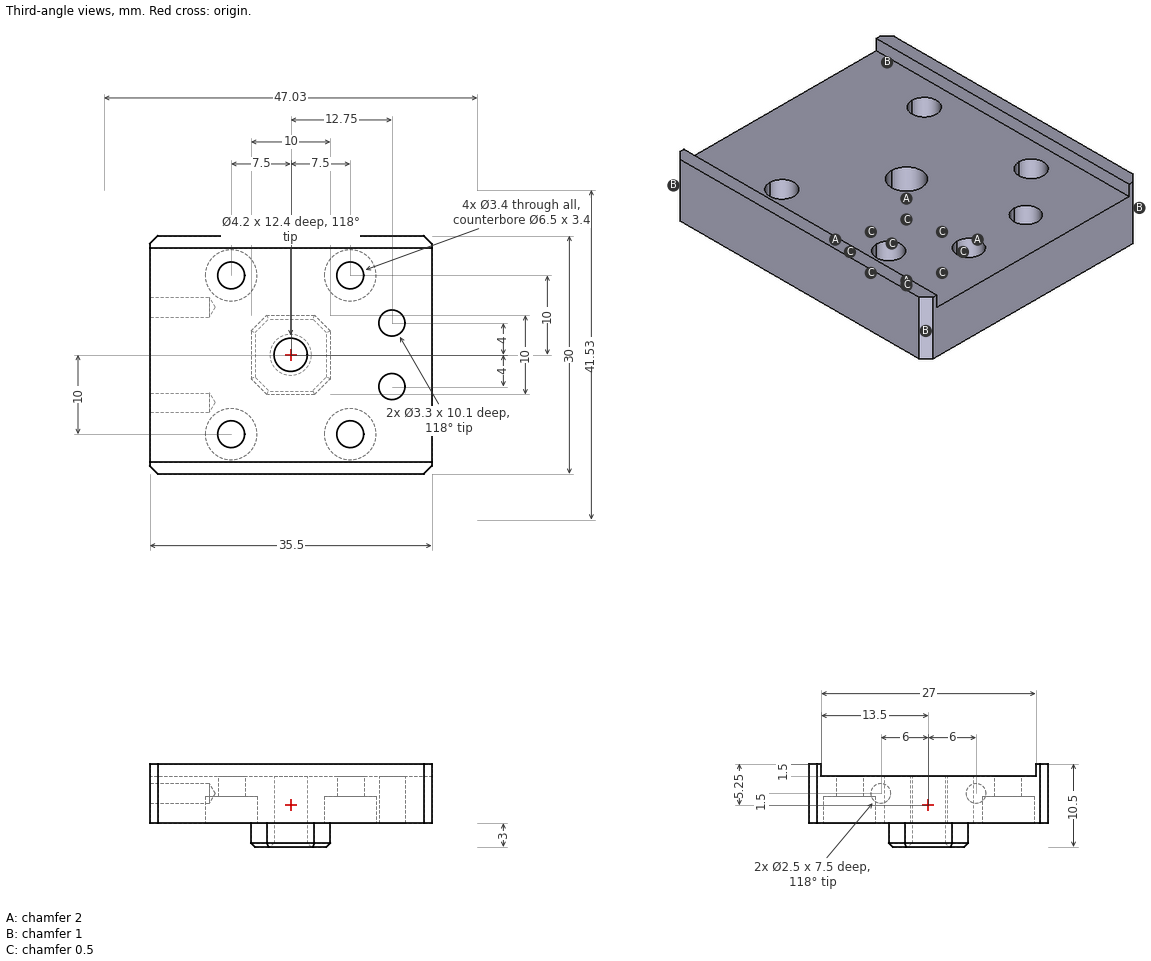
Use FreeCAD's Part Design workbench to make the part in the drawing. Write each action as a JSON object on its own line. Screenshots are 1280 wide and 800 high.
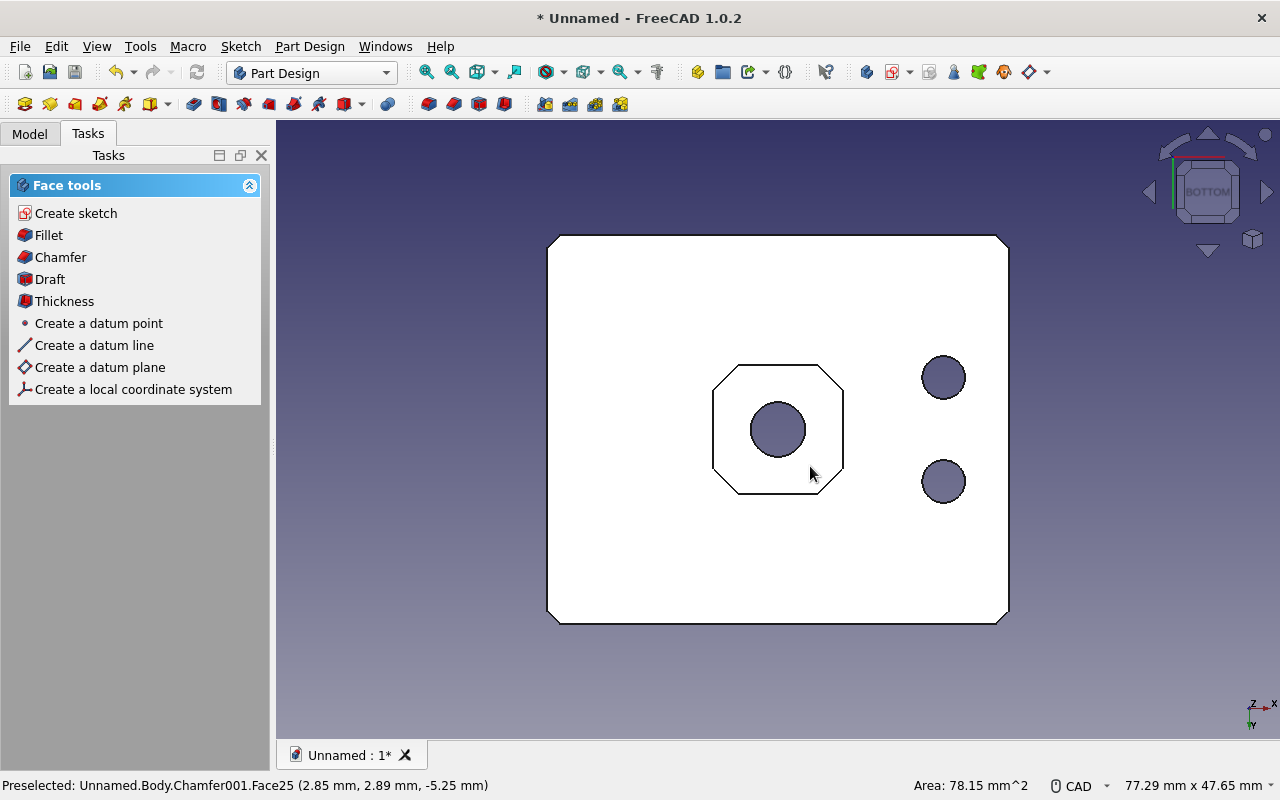
{"action": "left_click", "coordinate": [454, 104]}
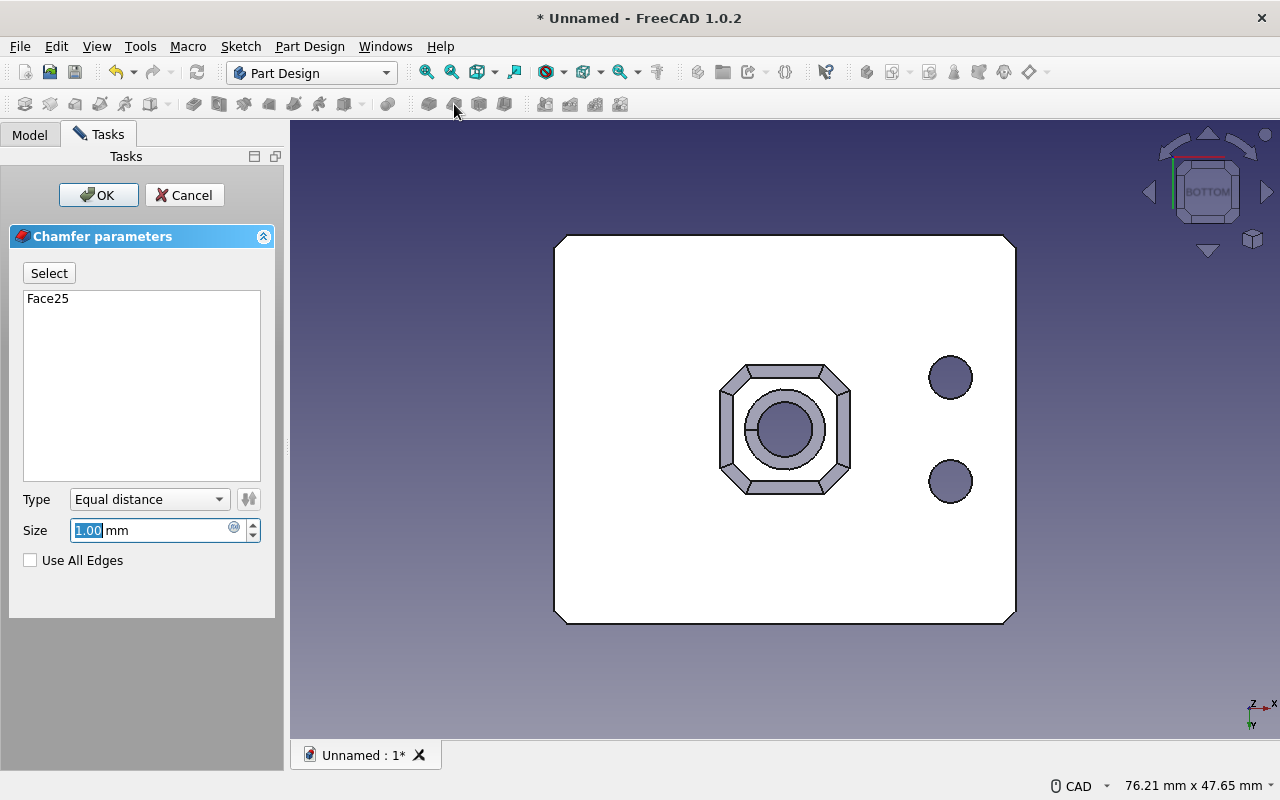
{"action": "type", "text": "0.5"}
{"action": "key", "text": "Tab"}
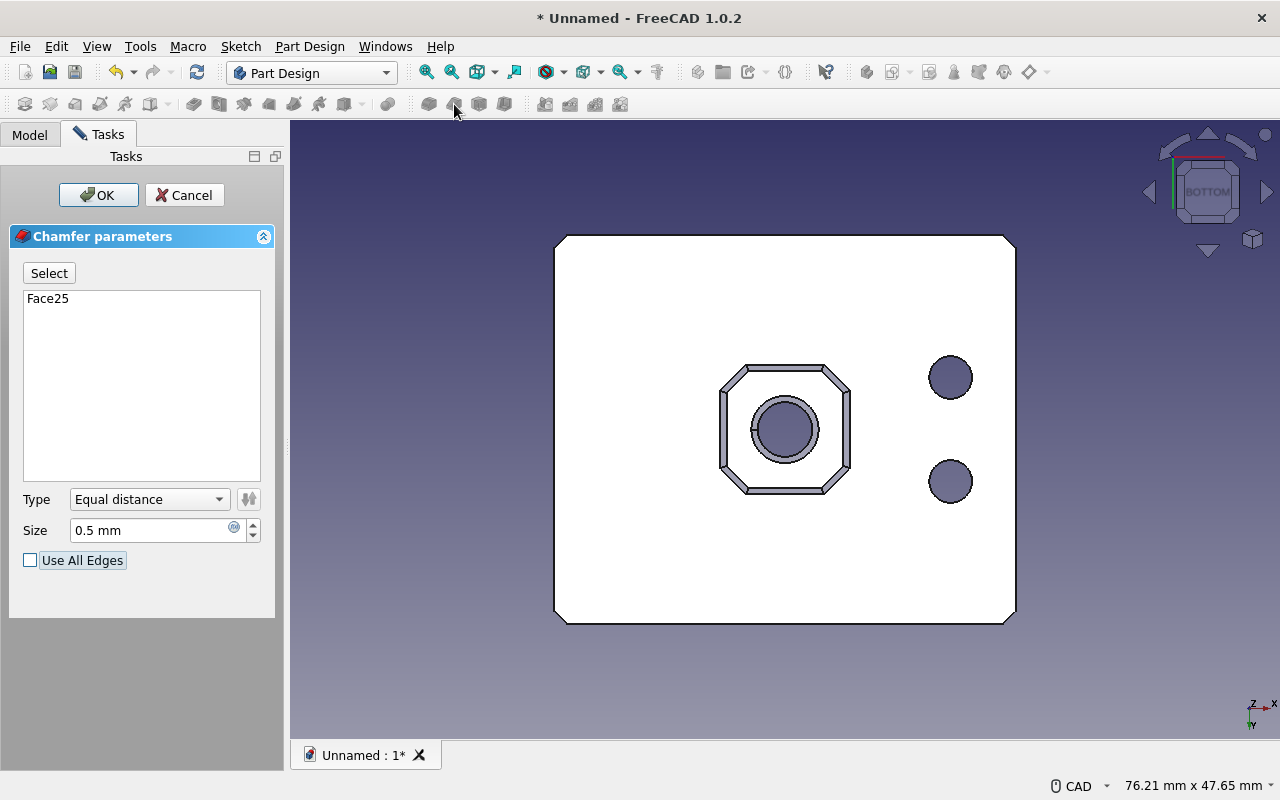
{"action": "left_click", "coordinate": [99, 195]}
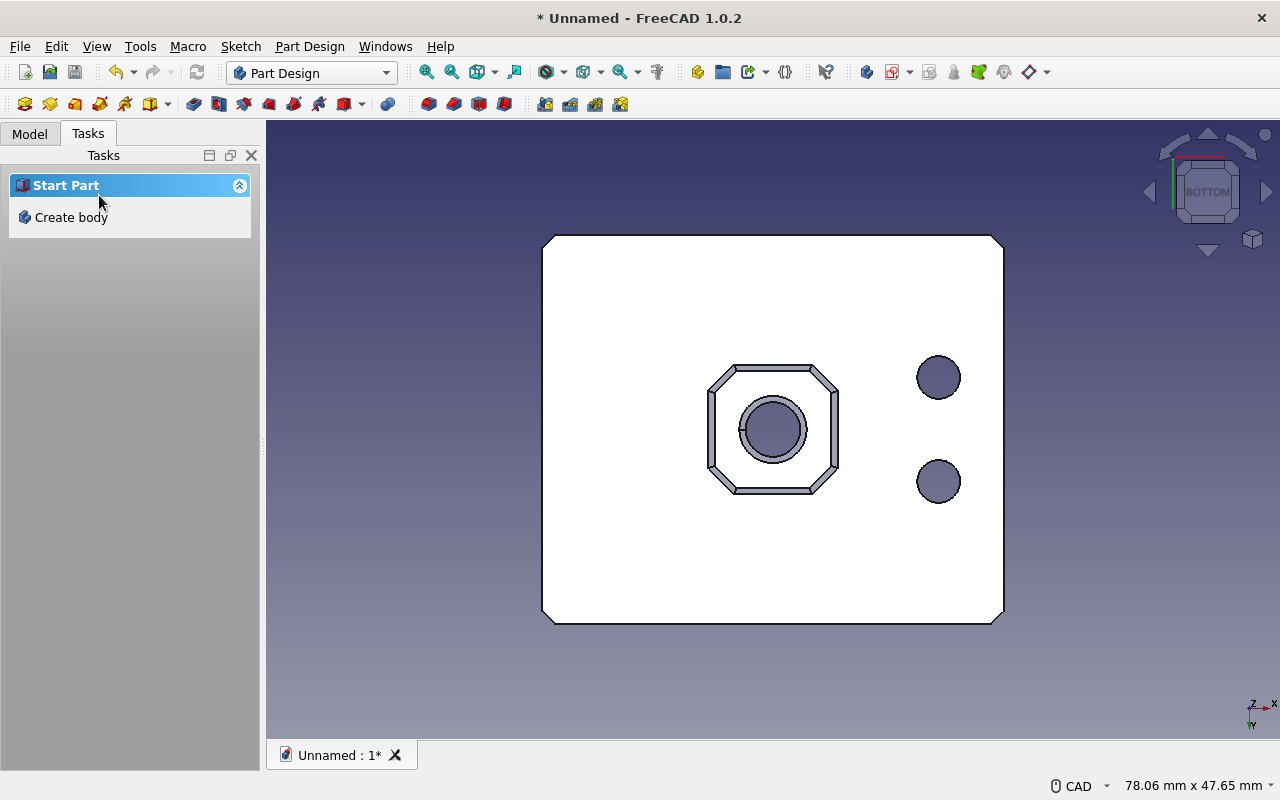
{"action": "left_click", "coordinate": [641, 317]}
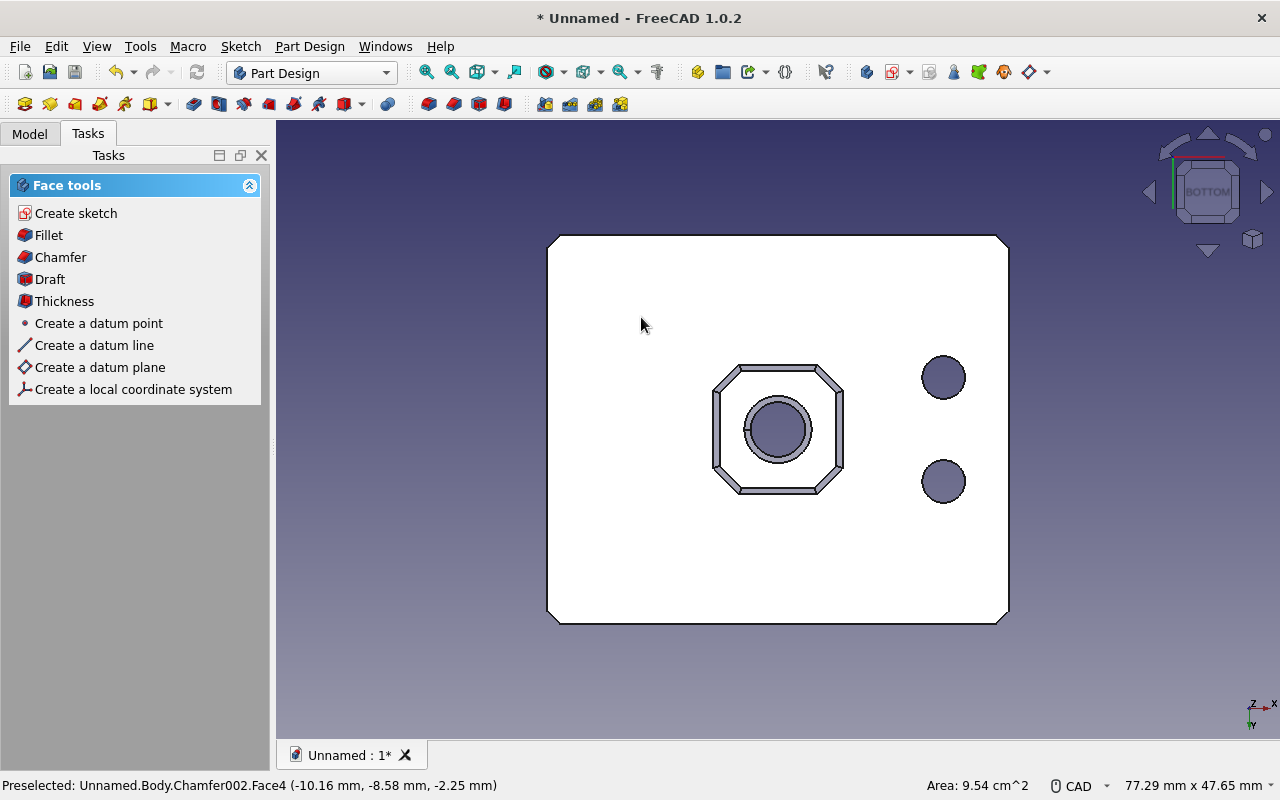
{"action": "left_click", "coordinate": [892, 72]}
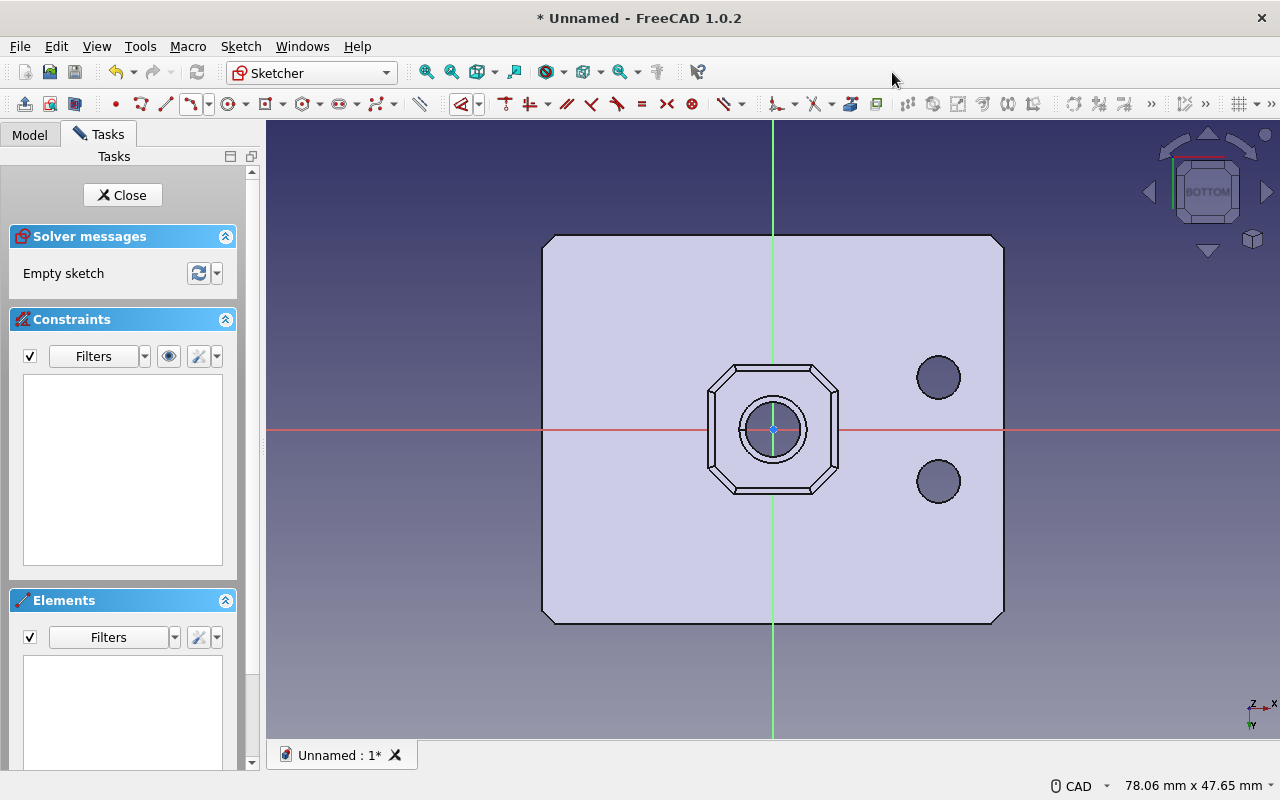
{"action": "key", "text": "q s"}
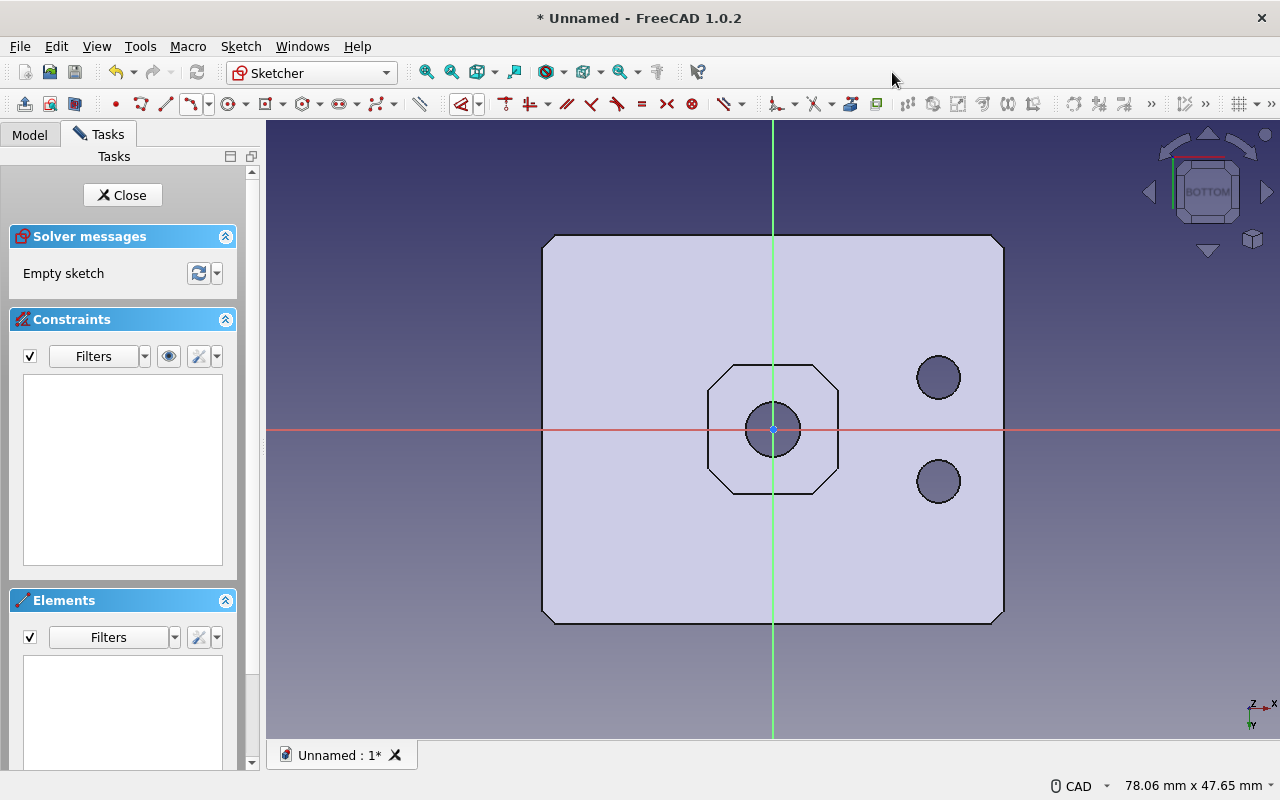
{"action": "key", "text": "g c"}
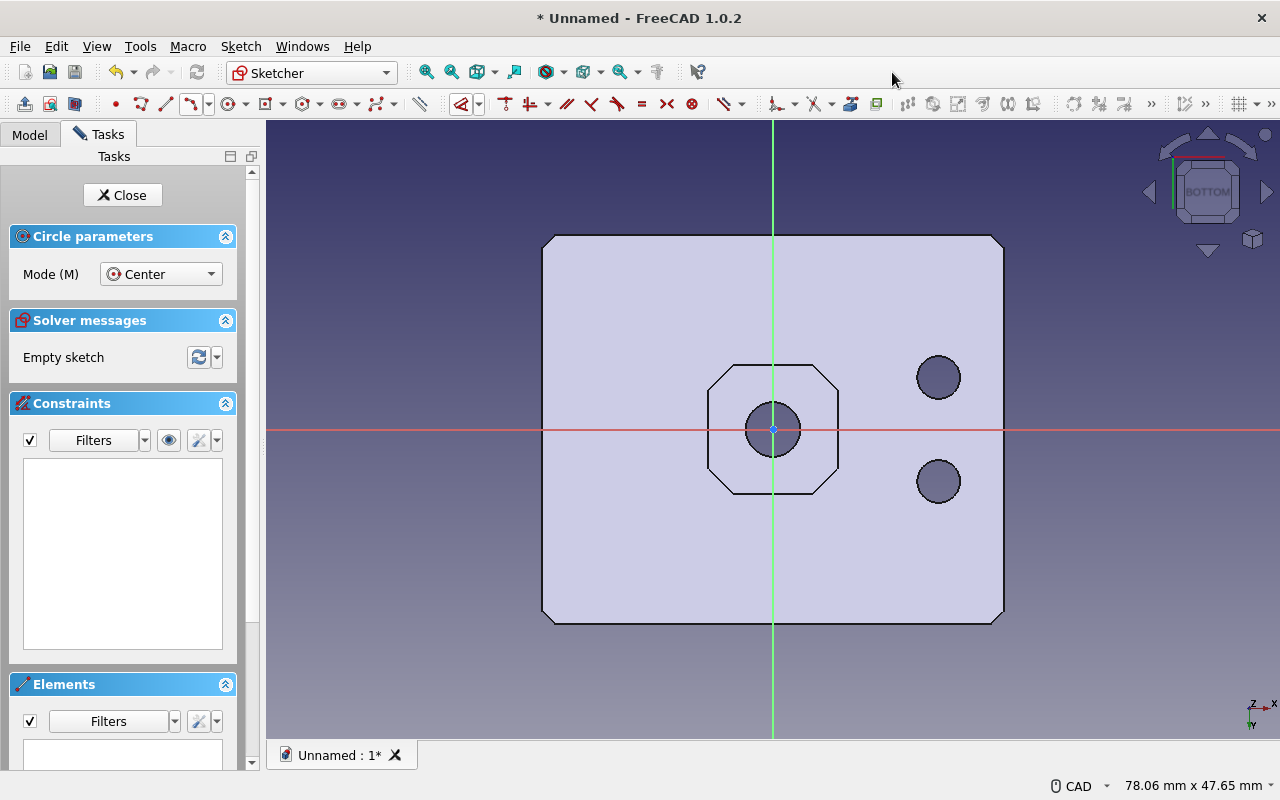
{"action": "left_click", "coordinate": [870, 559]}
{"action": "left_click", "coordinate": [886, 544]}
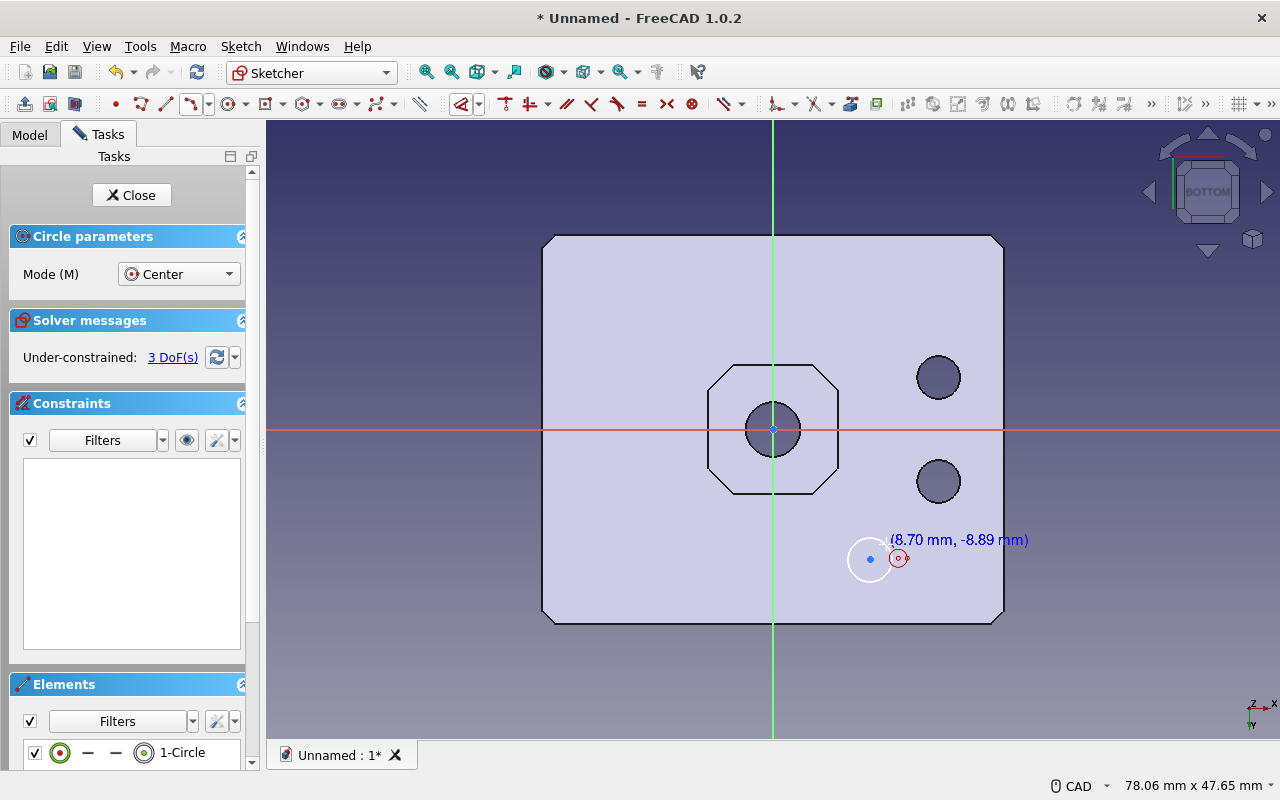
{"action": "left_click", "coordinate": [676, 559]}
{"action": "left_click", "coordinate": [691, 544]}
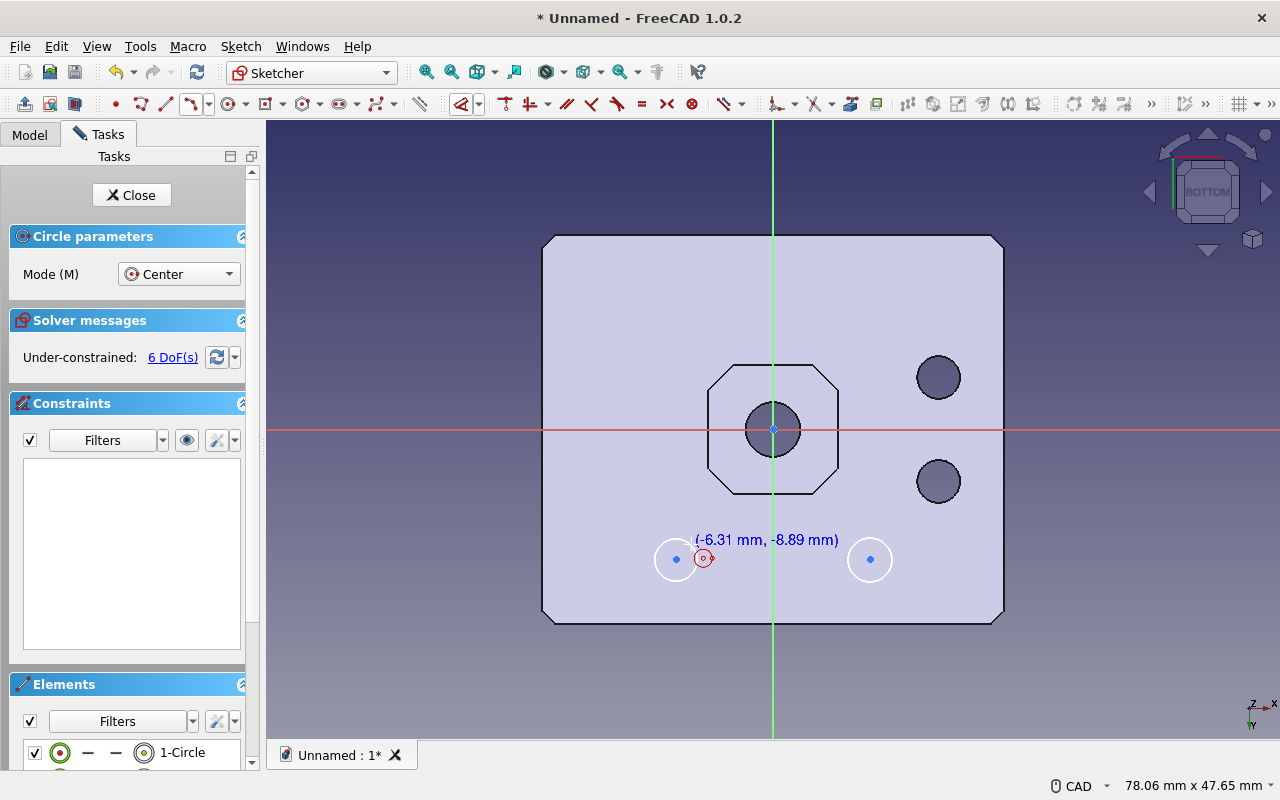
{"action": "left_click", "coordinate": [676, 300]}
{"action": "left_click", "coordinate": [691, 284]}